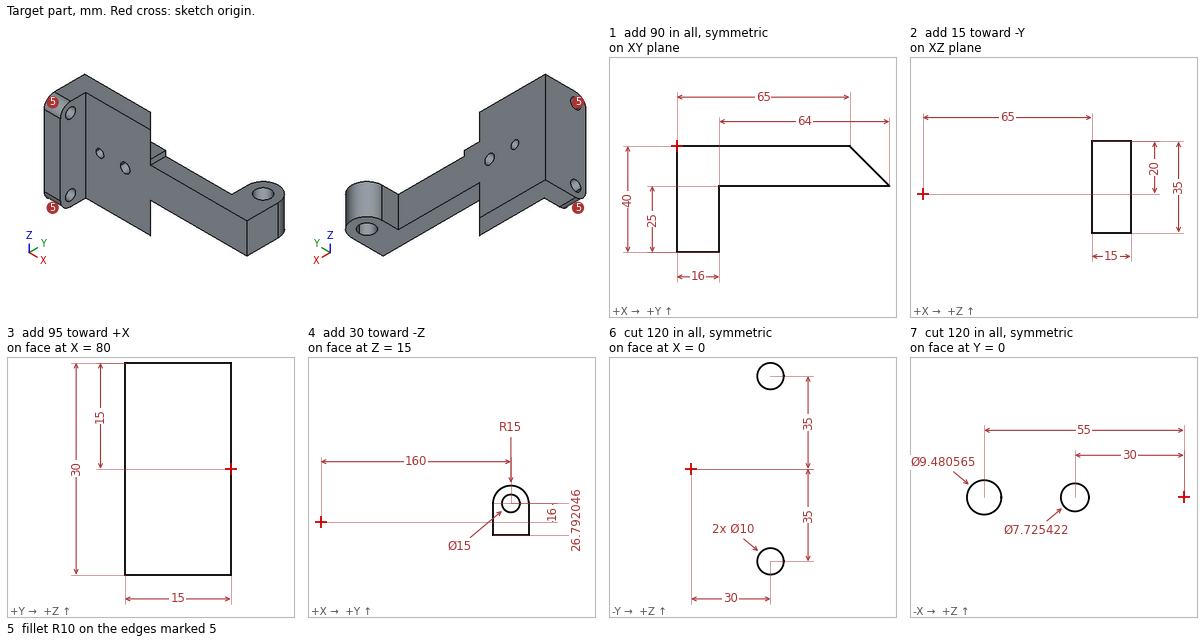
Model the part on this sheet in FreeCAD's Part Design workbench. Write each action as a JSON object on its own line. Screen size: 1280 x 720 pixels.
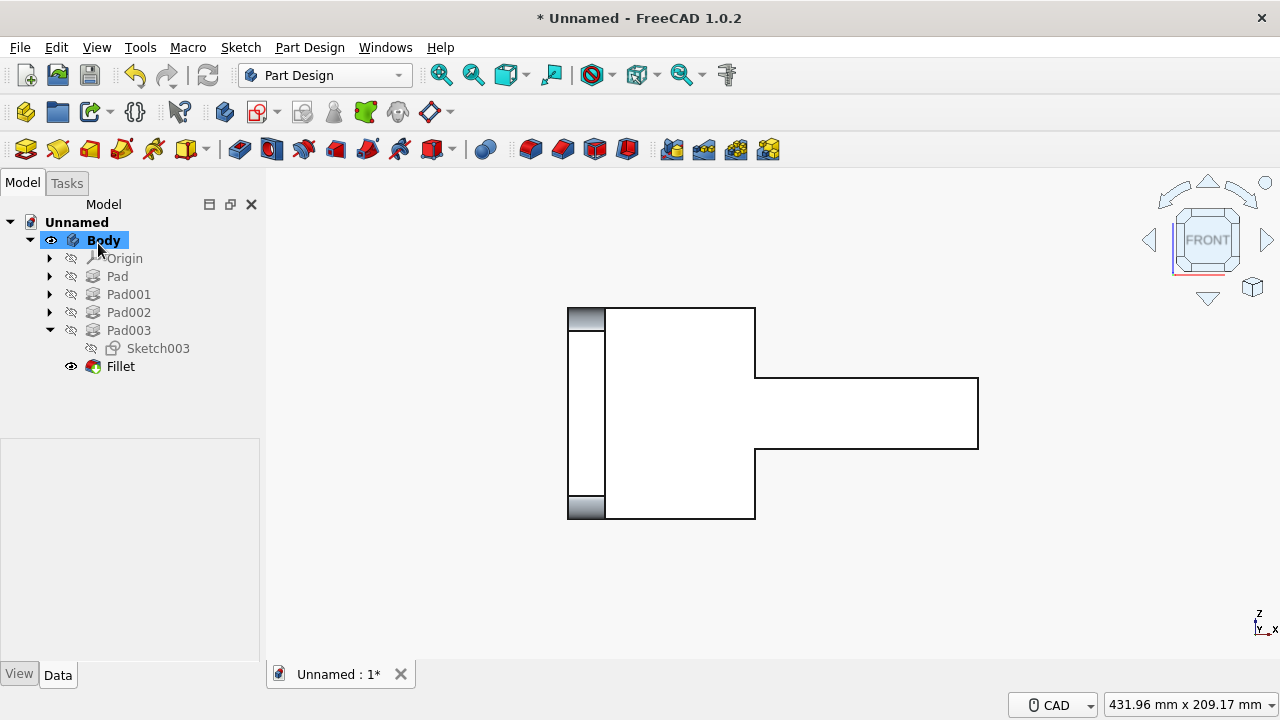
{"action": "left_click", "coordinate": [442, 76]}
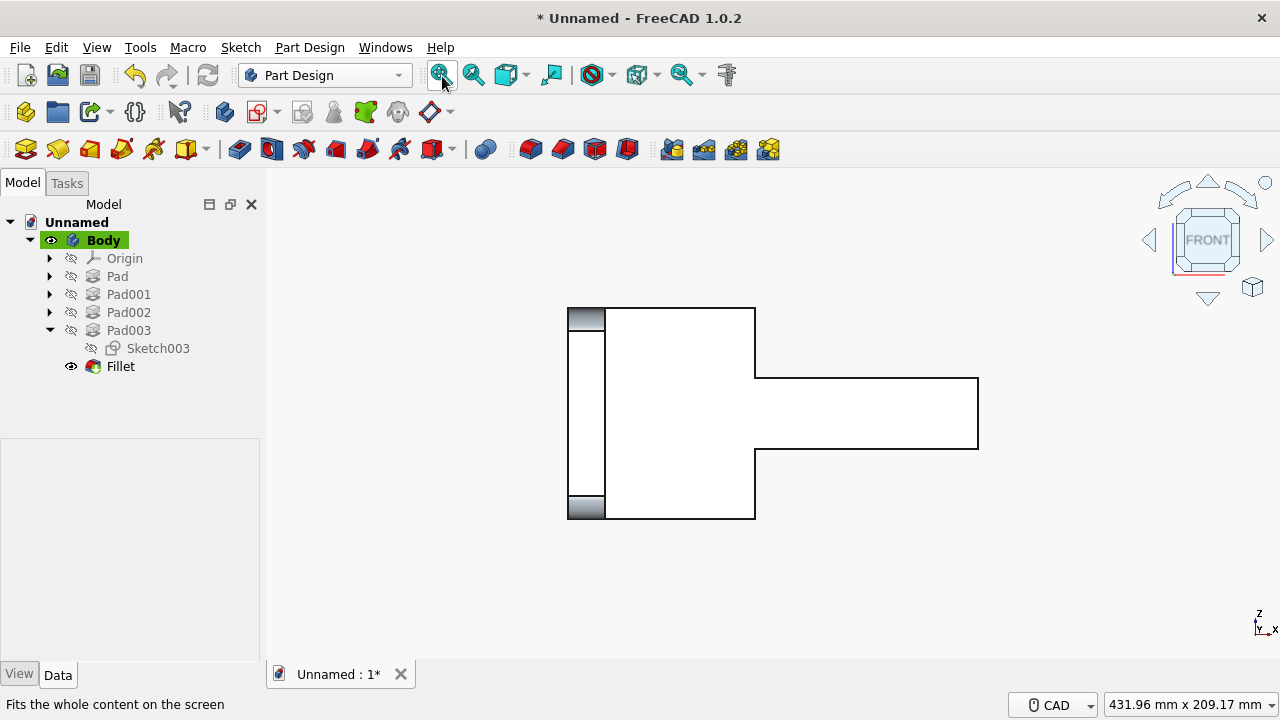
{"action": "key", "text": "6"}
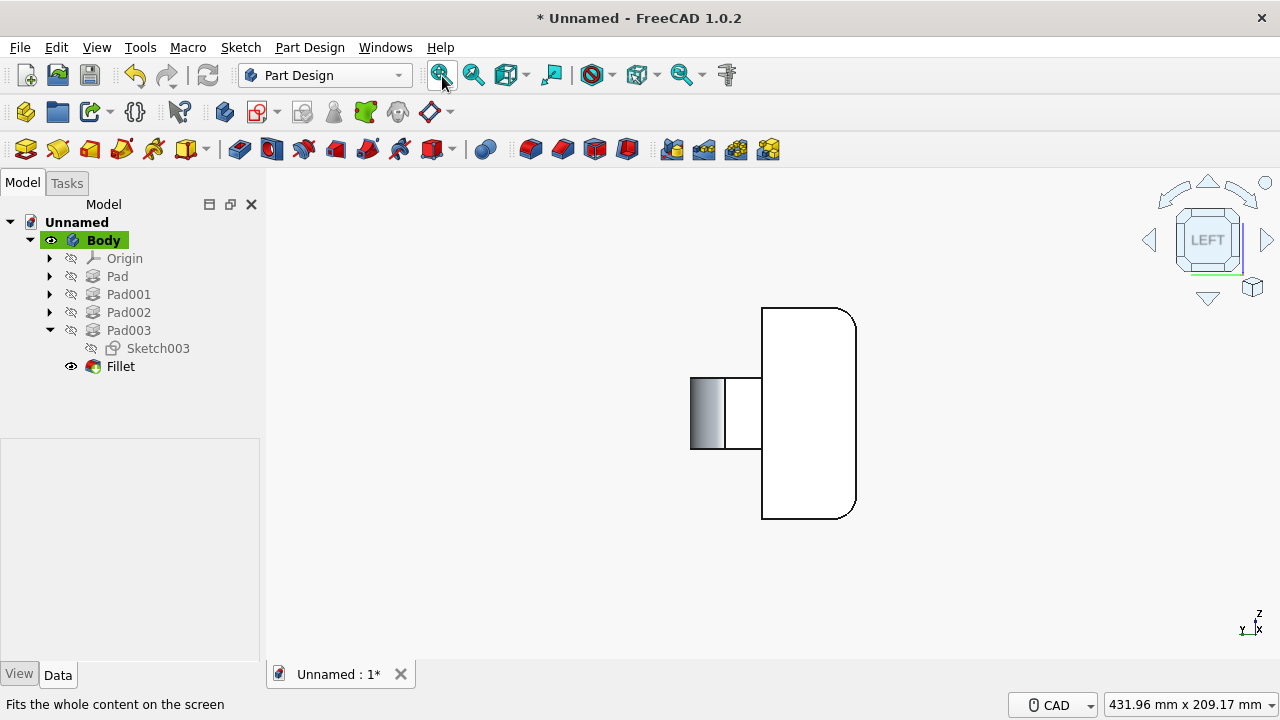
{"action": "key", "text": "v f"}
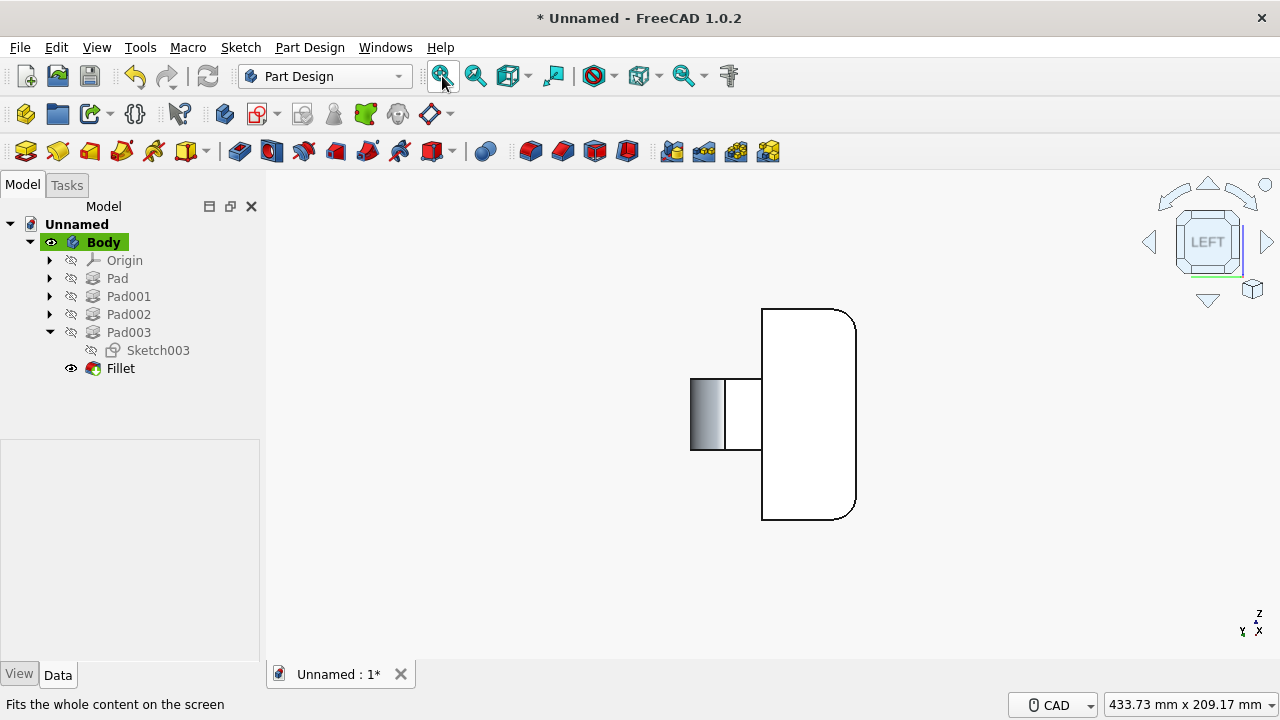
{"action": "left_click", "coordinate": [809, 383]}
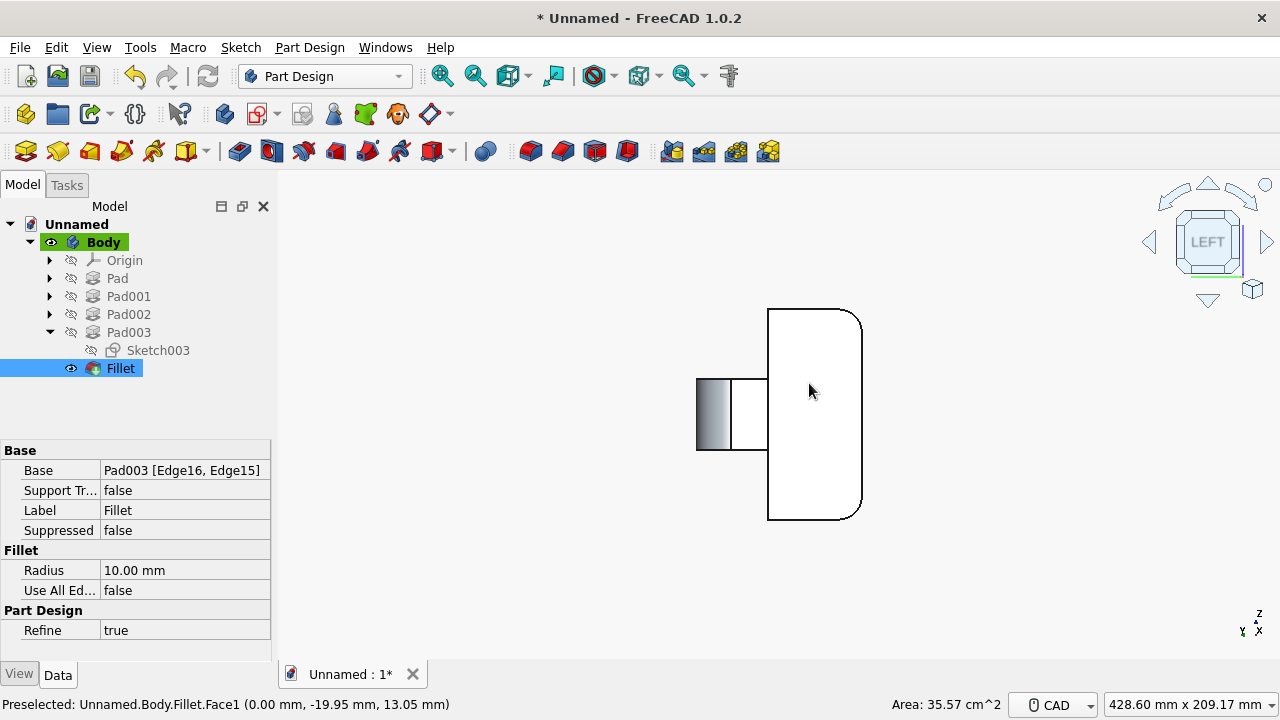
{"action": "left_click", "coordinate": [258, 114]}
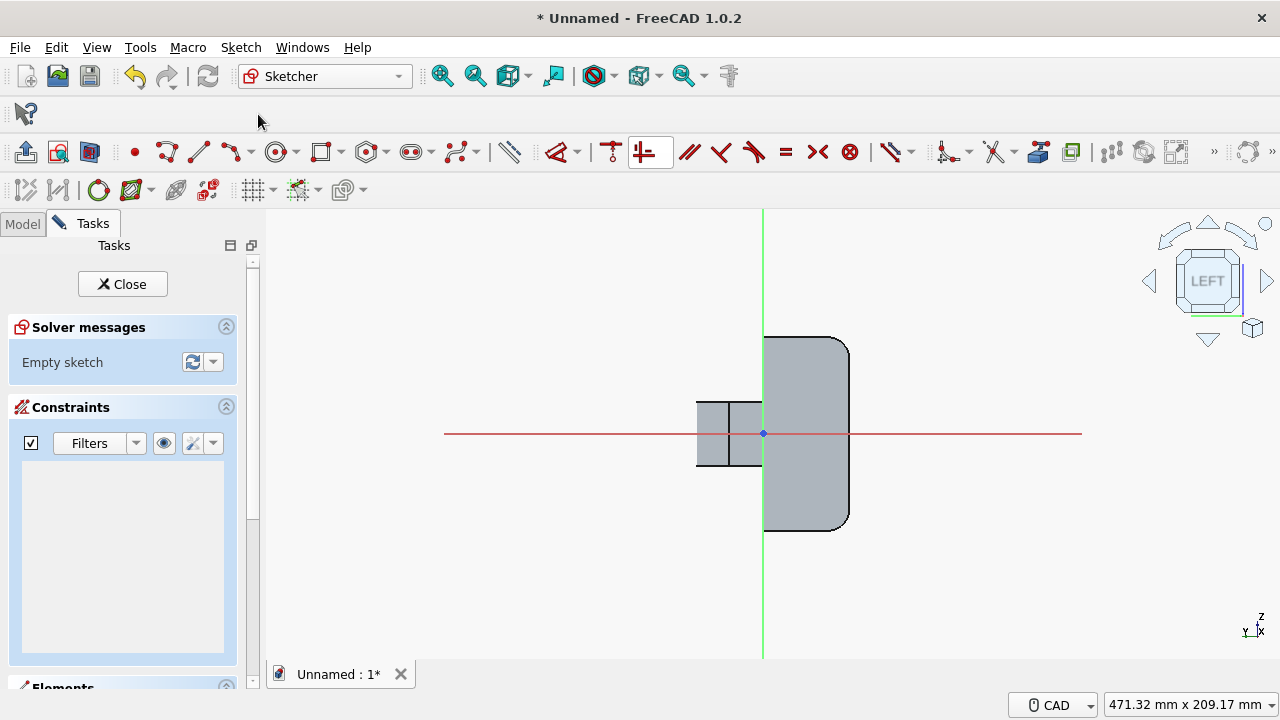
{"action": "scroll", "coordinate": [997, 434], "scroll_direction": "up", "scroll_amount": 2}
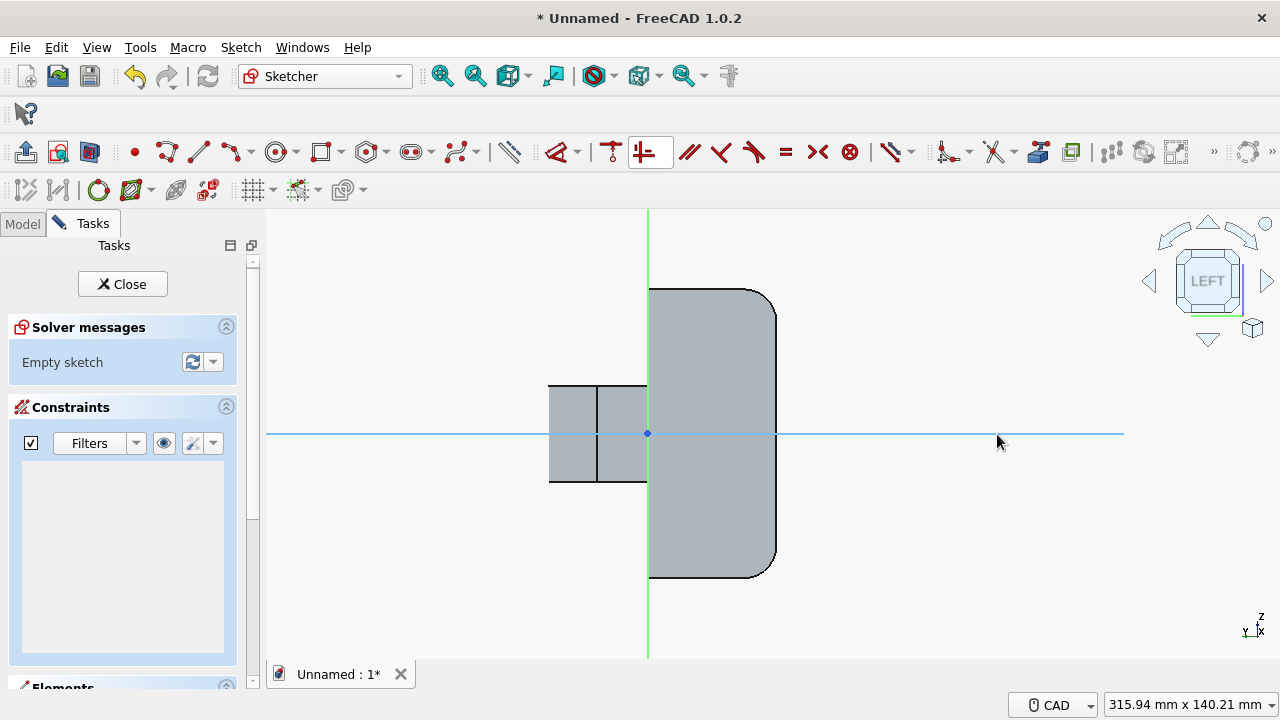
{"action": "left_click", "coordinate": [276, 152]}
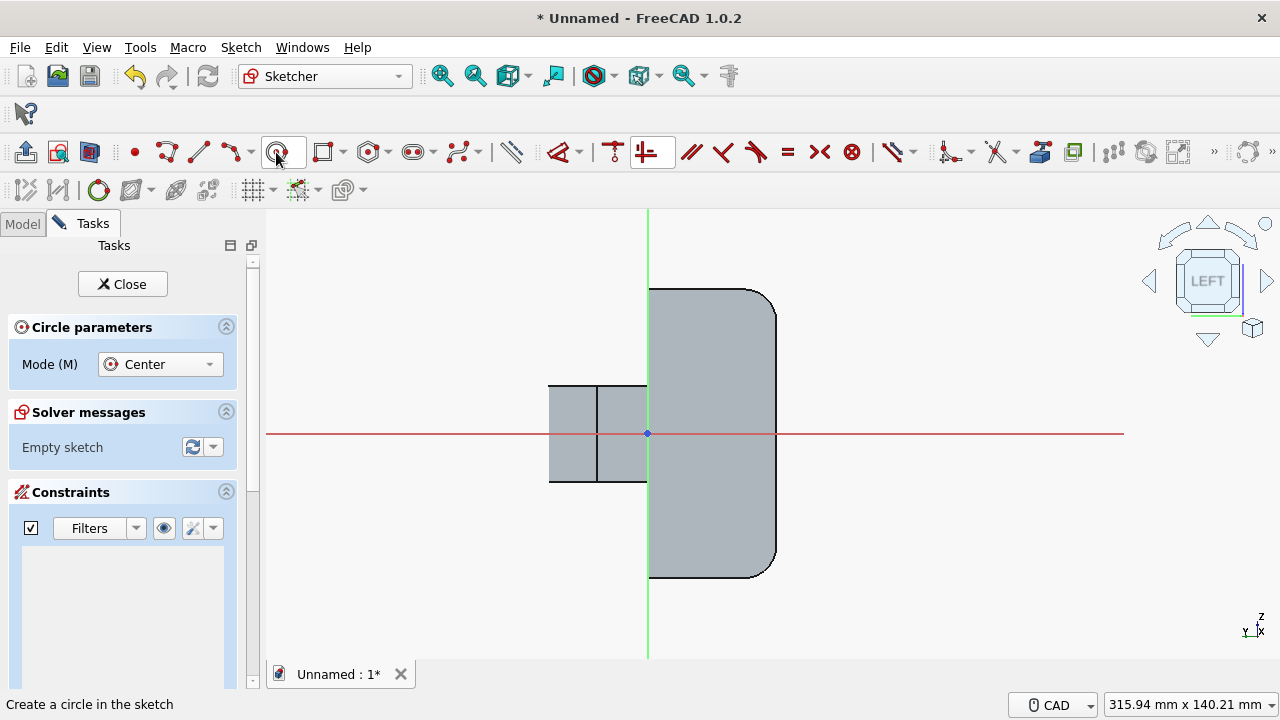
{"action": "scroll", "coordinate": [744, 546], "scroll_direction": "up", "scroll_amount": 2}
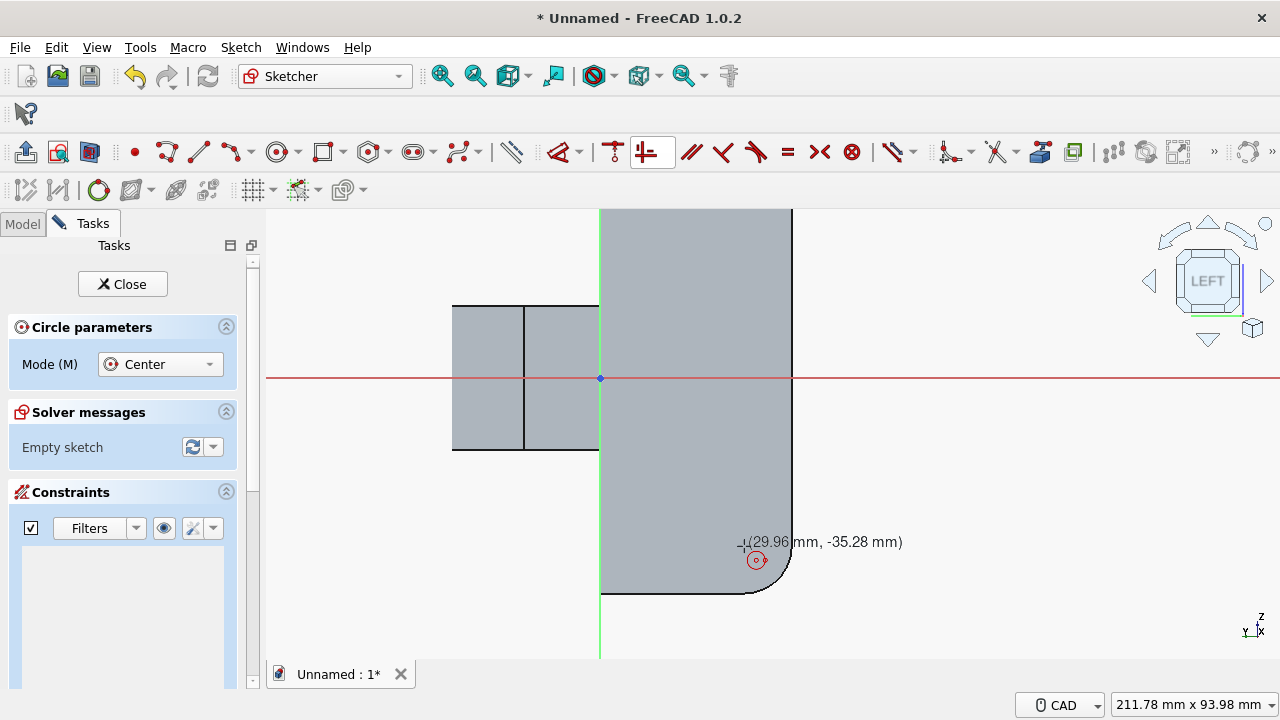
{"action": "left_click", "coordinate": [744, 546]}
{"action": "mouse_move", "coordinate": [761, 529]}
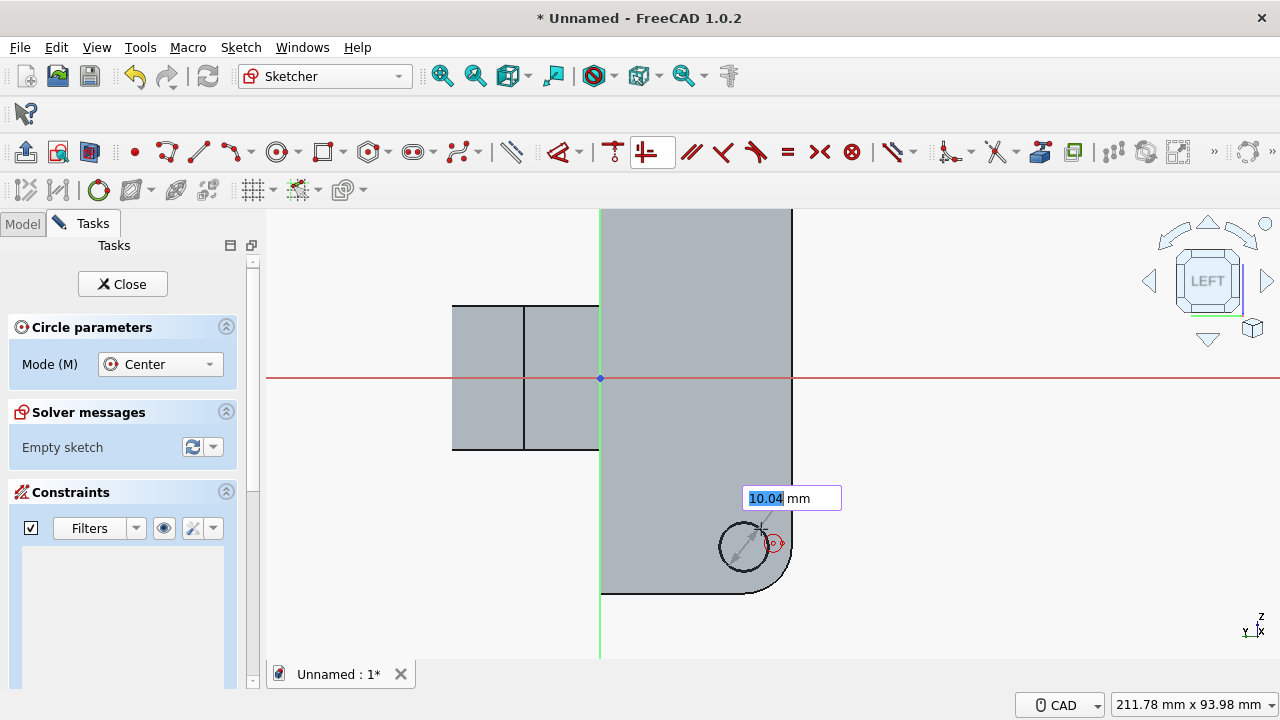
{"action": "type", "text": "10"}
{"action": "key", "text": "Return"}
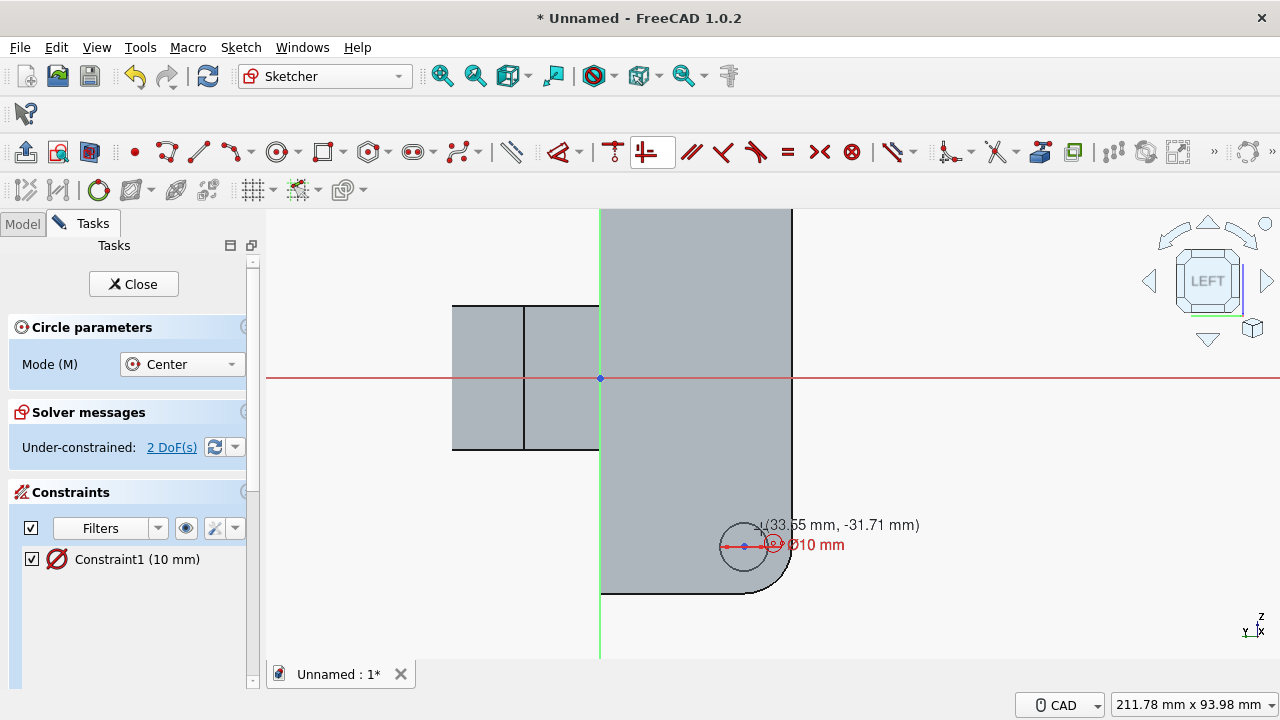
{"action": "scroll", "coordinate": [746, 547], "scroll_direction": "down", "scroll_amount": 2}